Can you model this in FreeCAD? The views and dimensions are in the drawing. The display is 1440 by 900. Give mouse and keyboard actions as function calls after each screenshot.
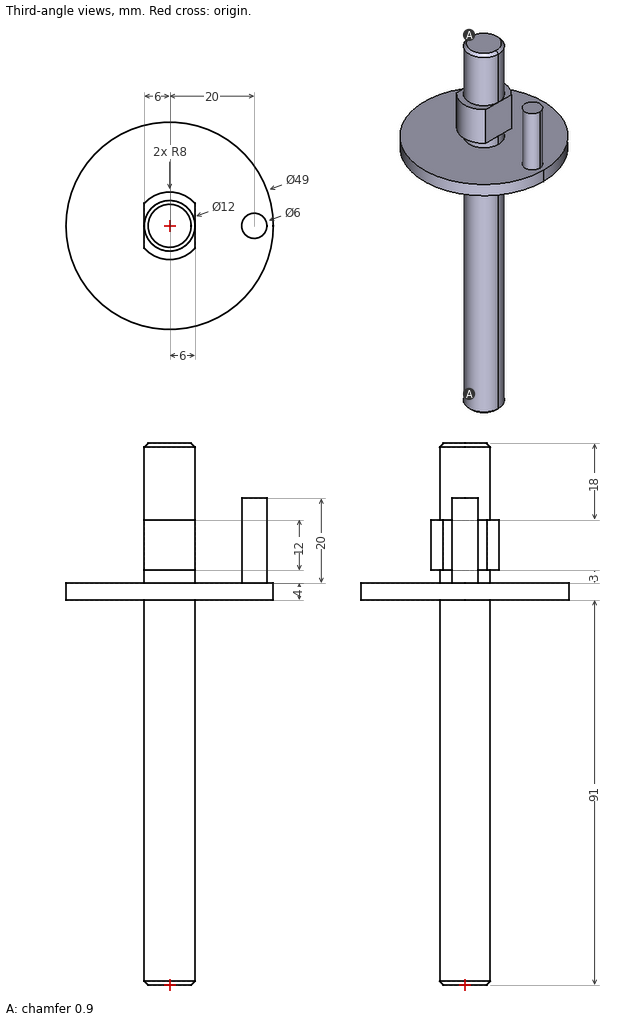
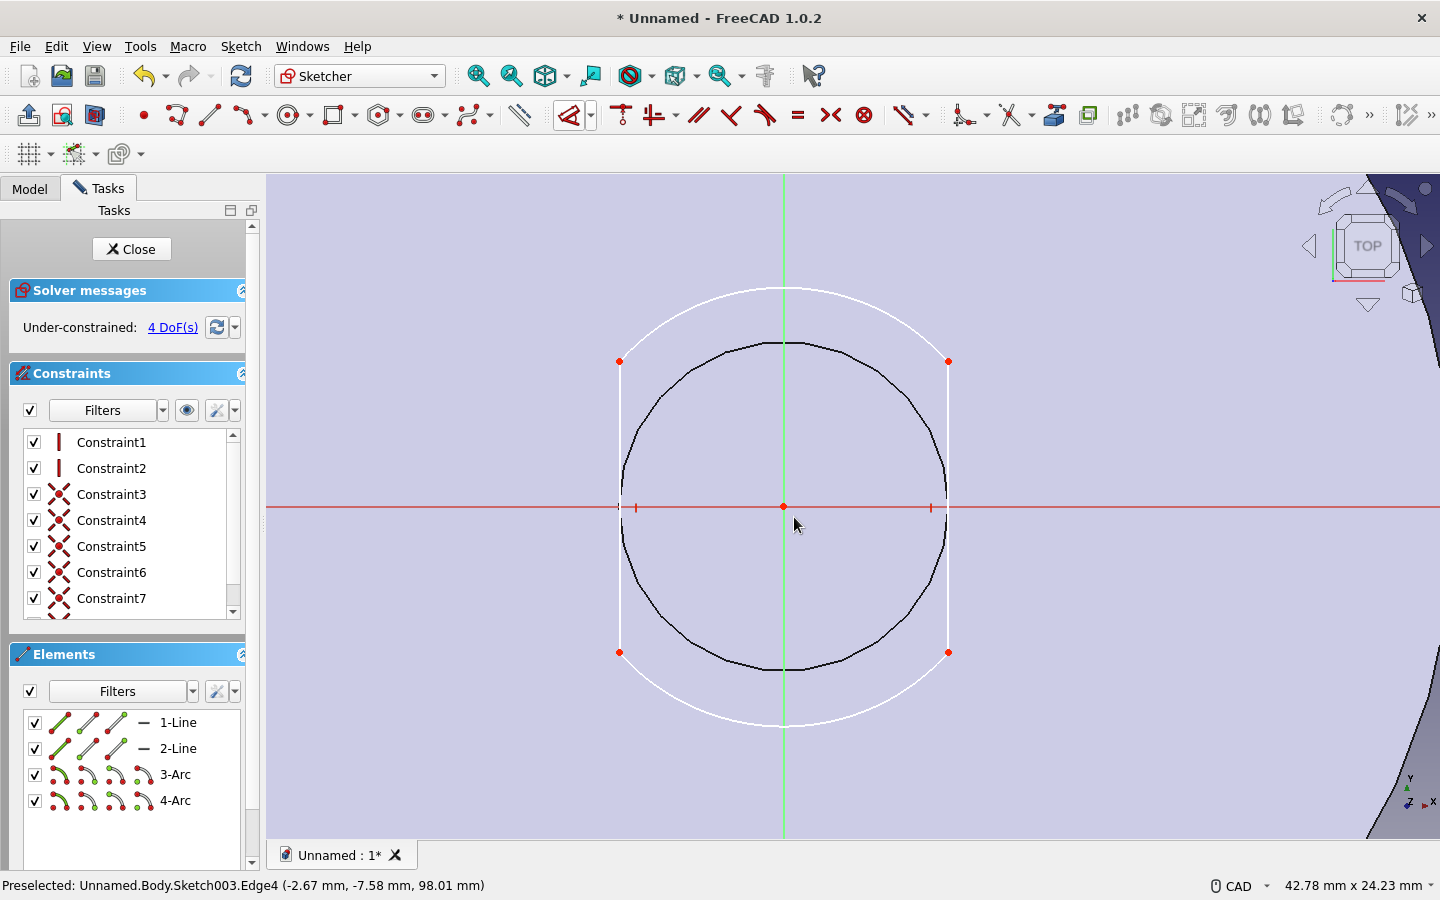
click(857, 300)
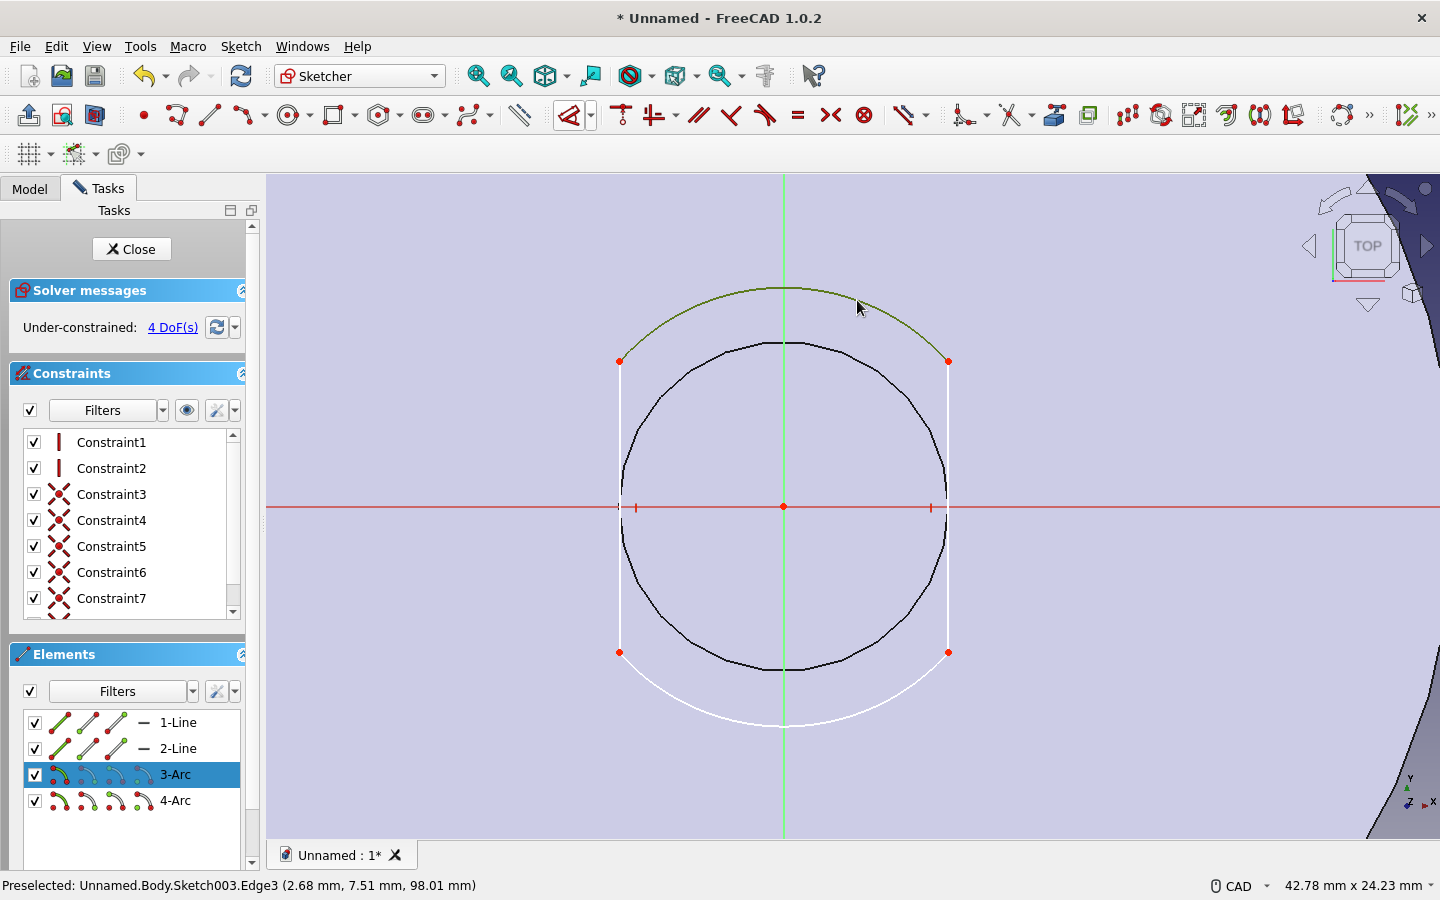
click(711, 714)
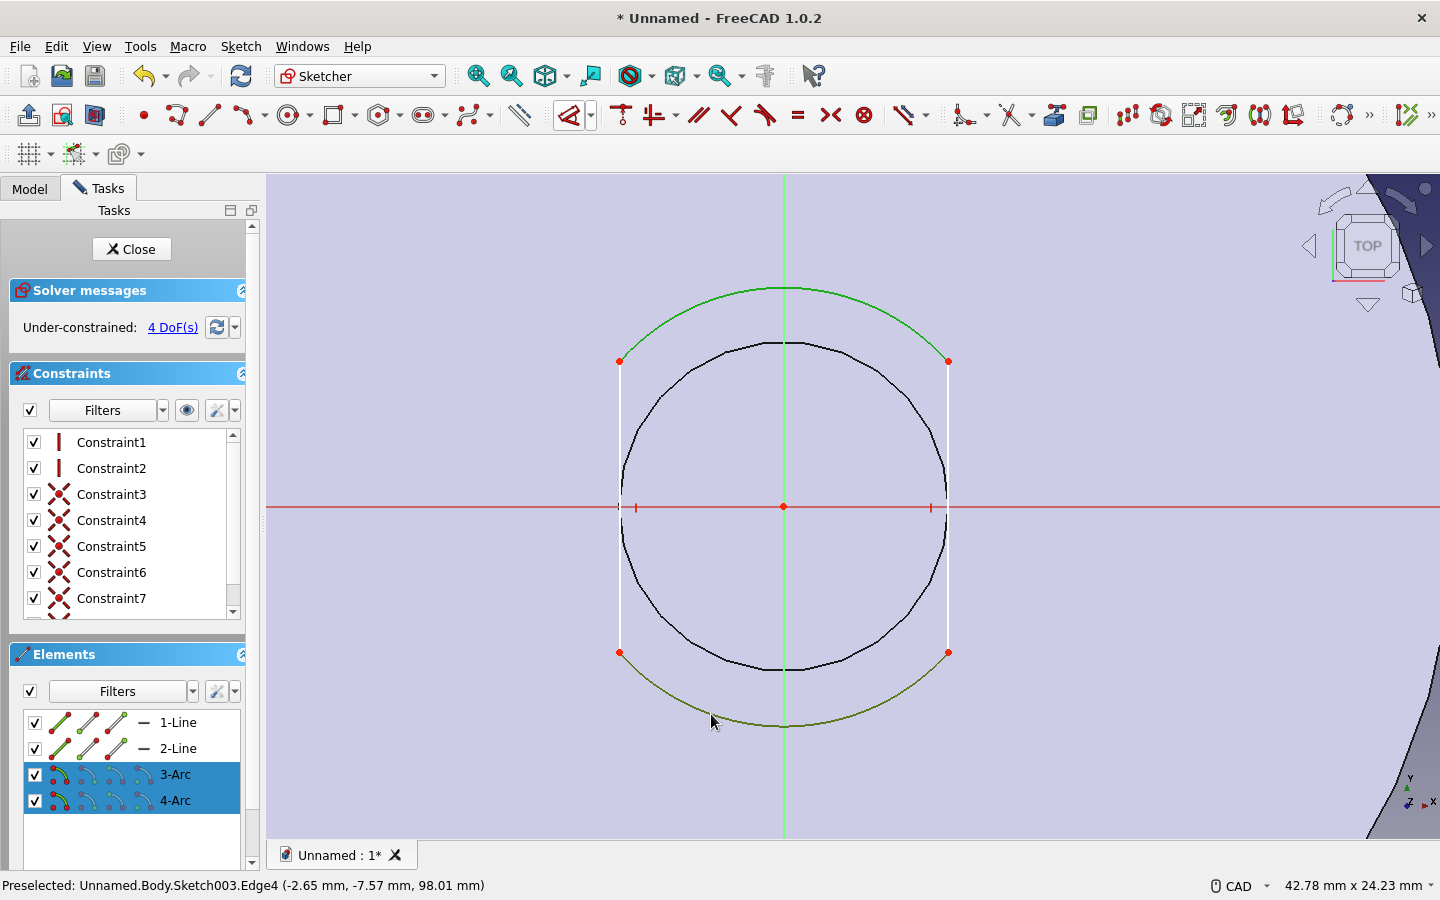
key(e)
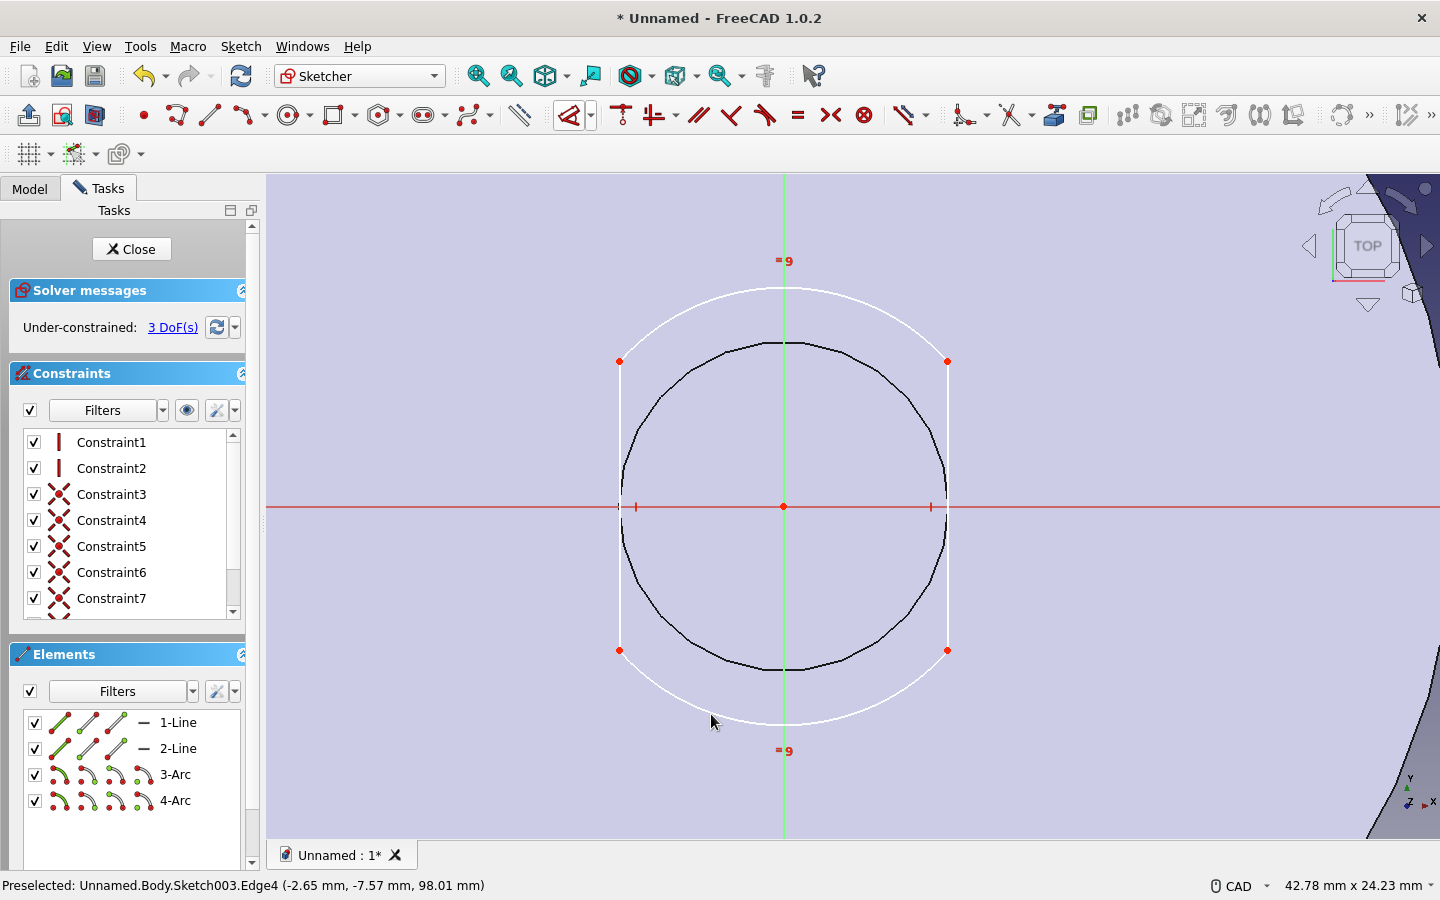
click(857, 300)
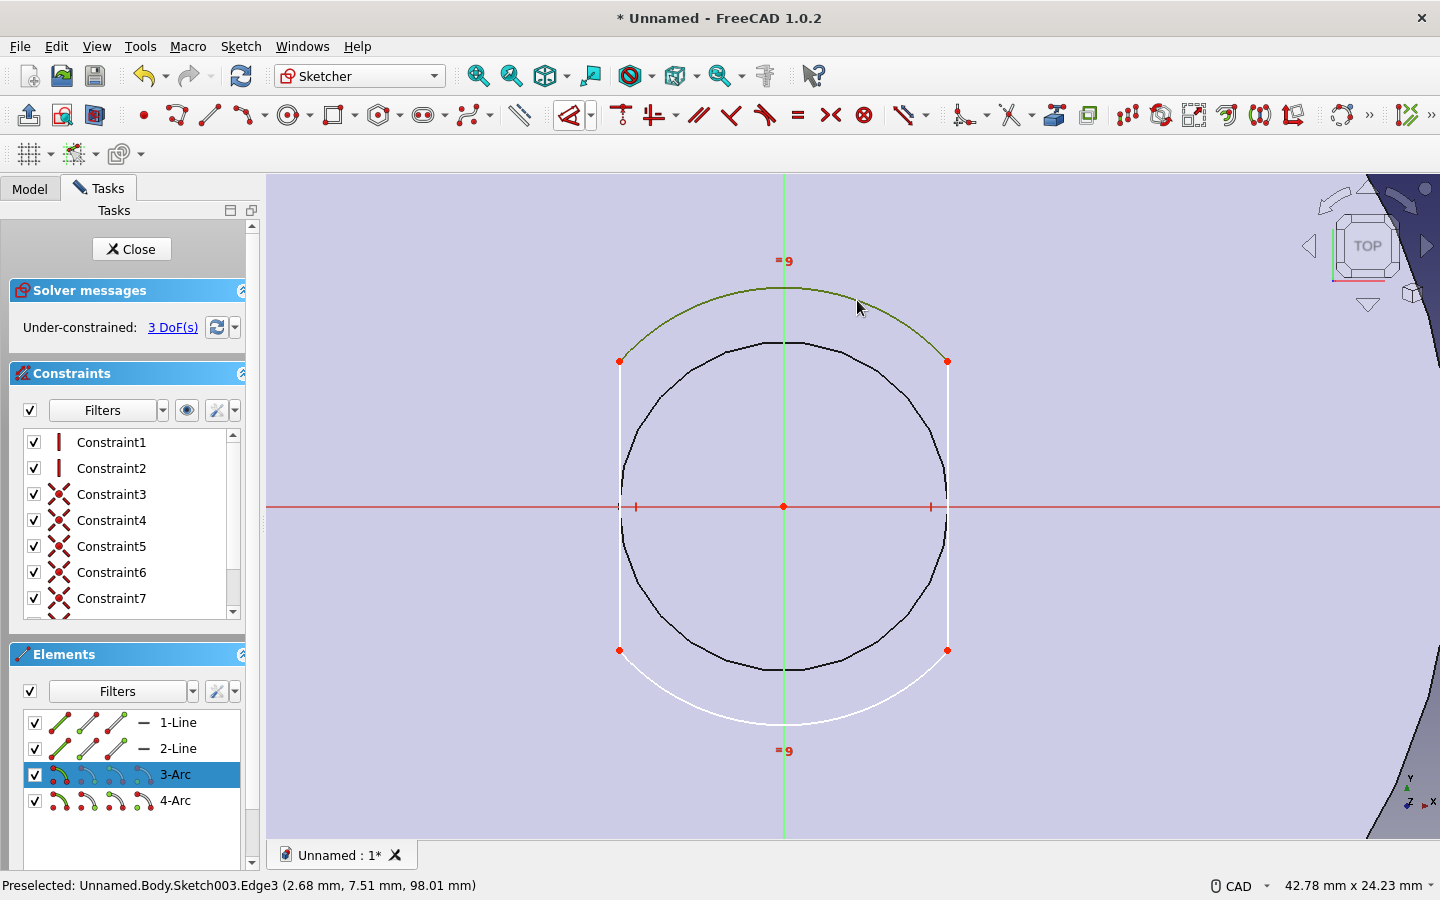
key(k)
key(r)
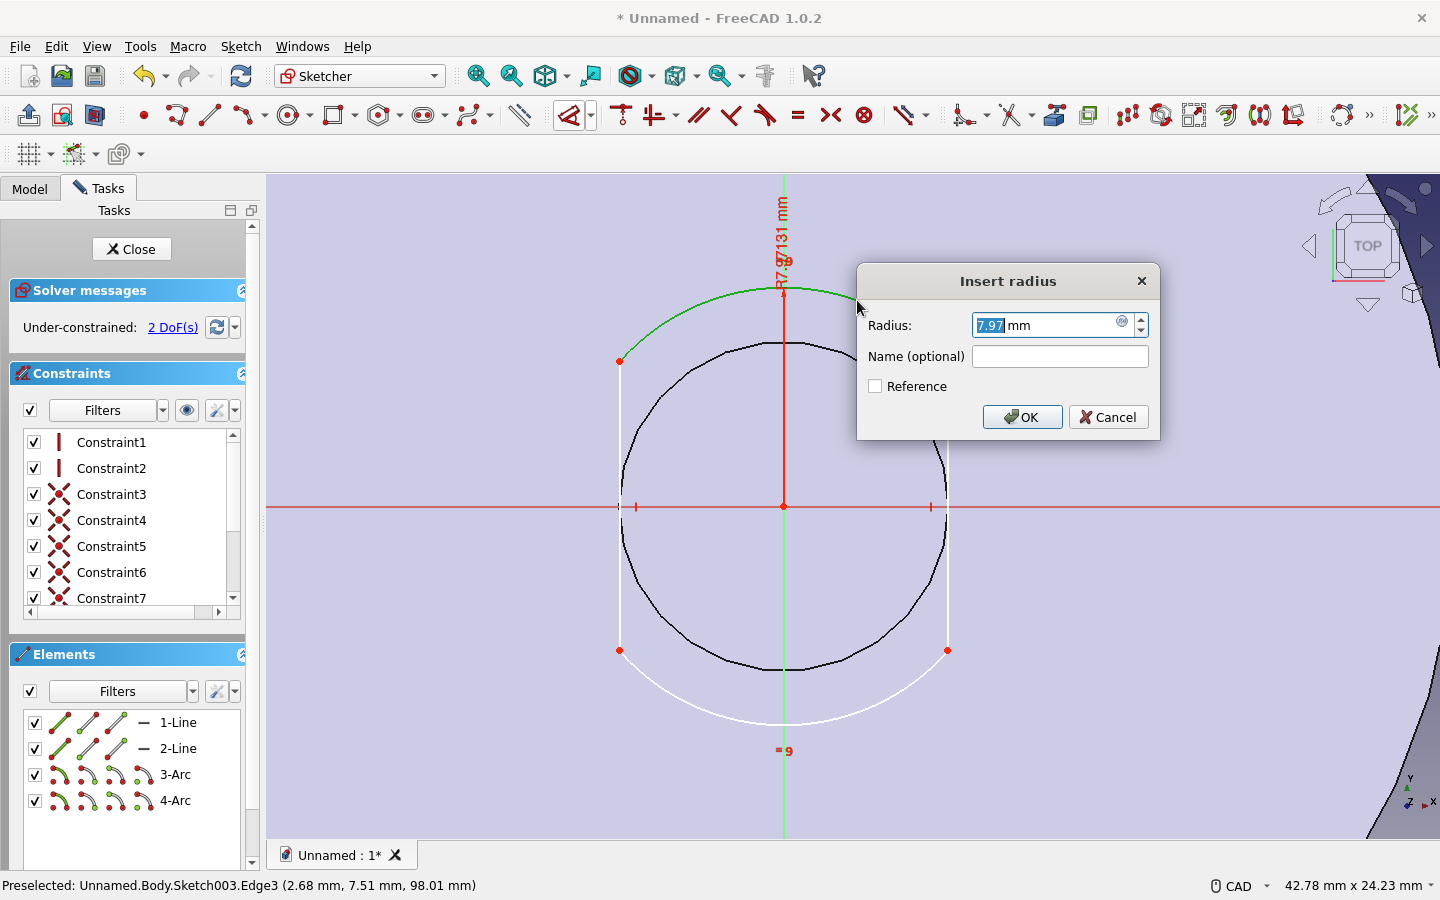
text(8)
key(Return)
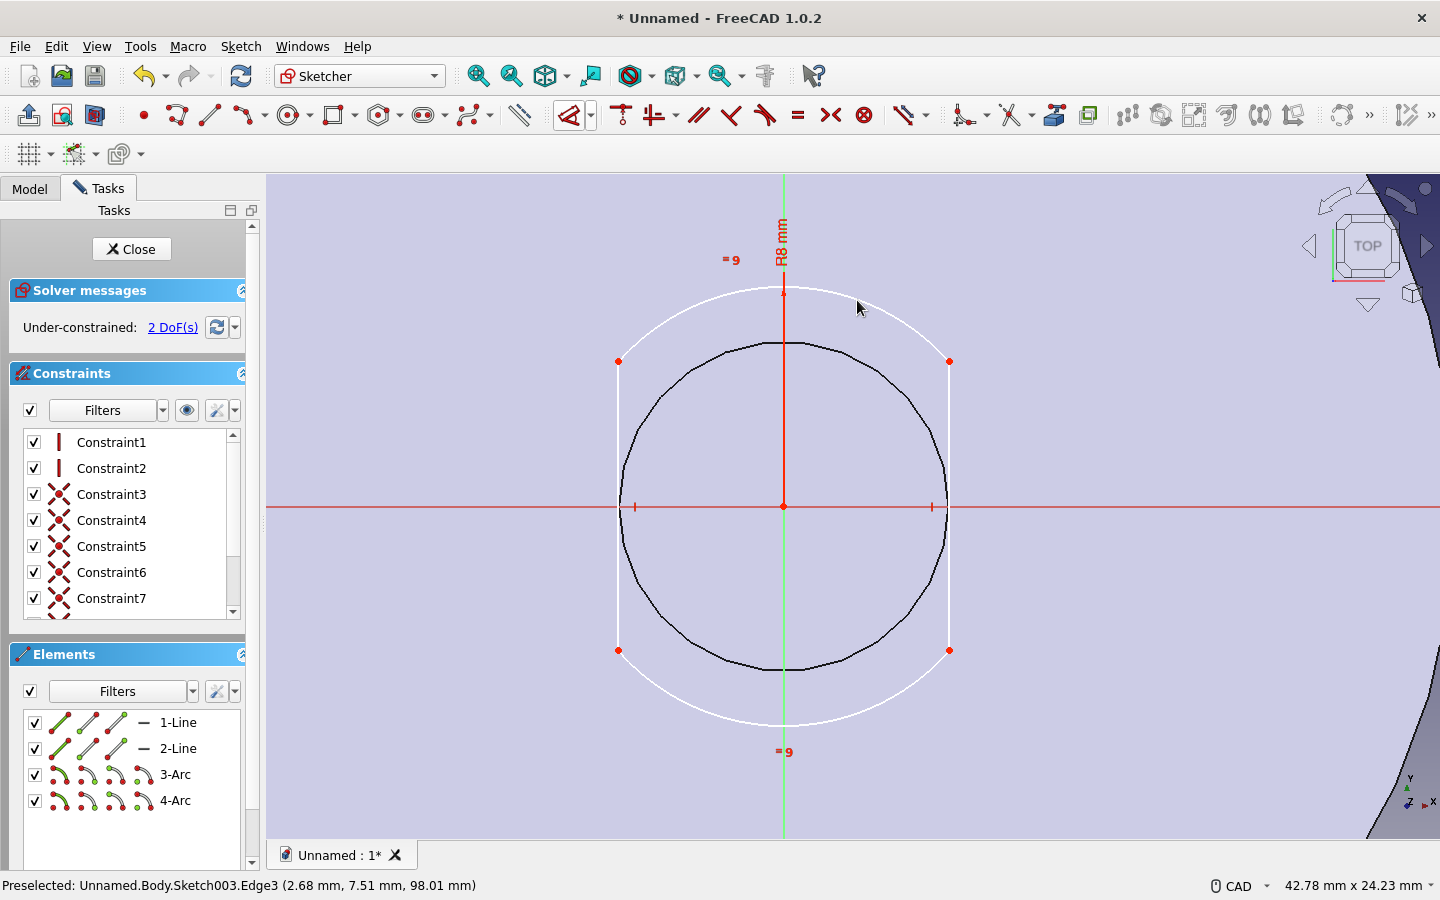
click(949, 651)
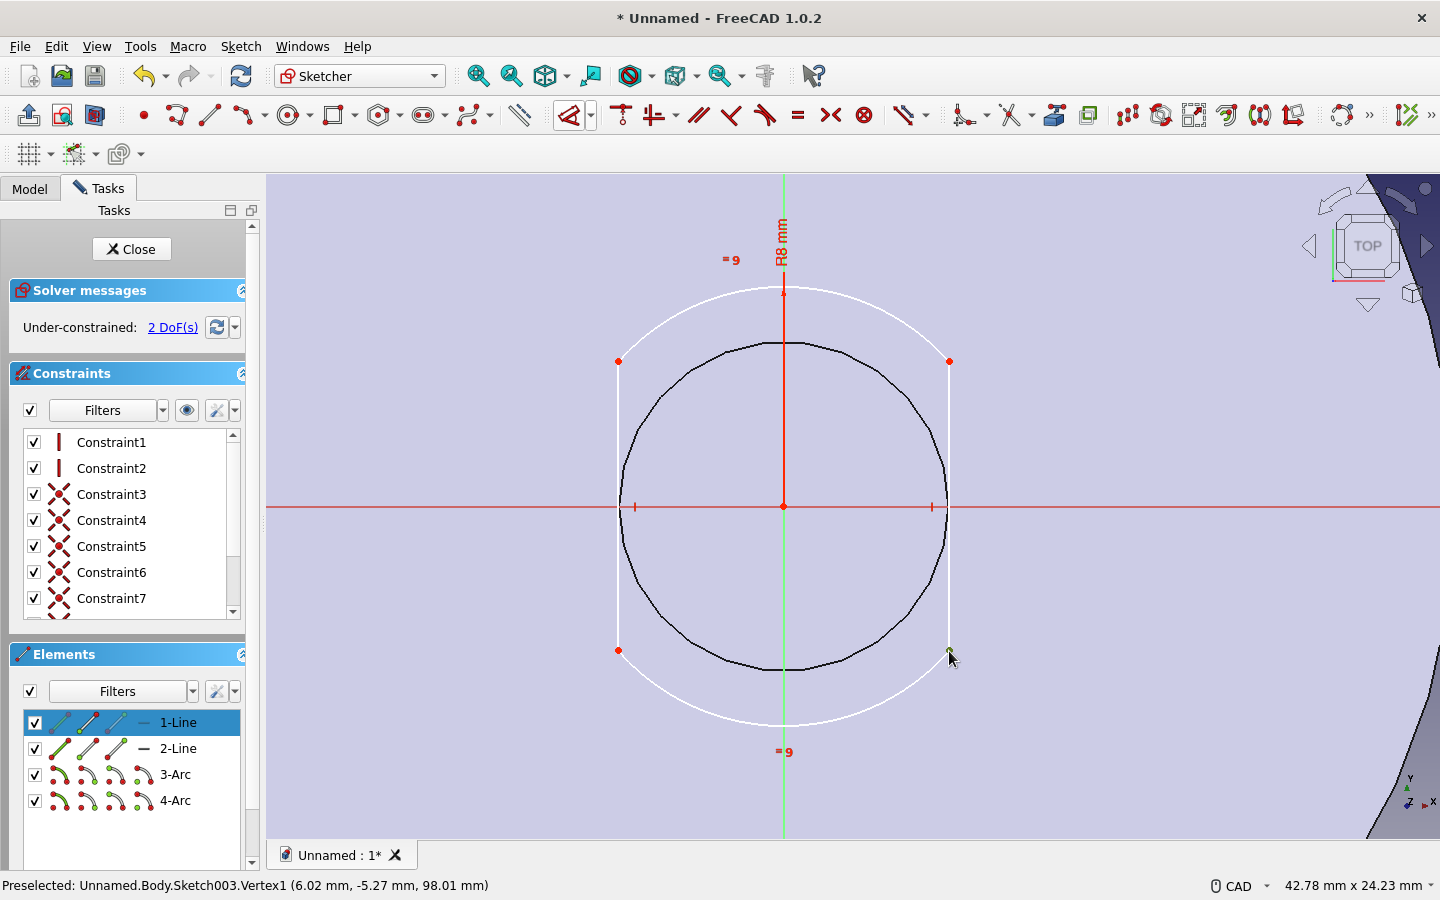
key(l)